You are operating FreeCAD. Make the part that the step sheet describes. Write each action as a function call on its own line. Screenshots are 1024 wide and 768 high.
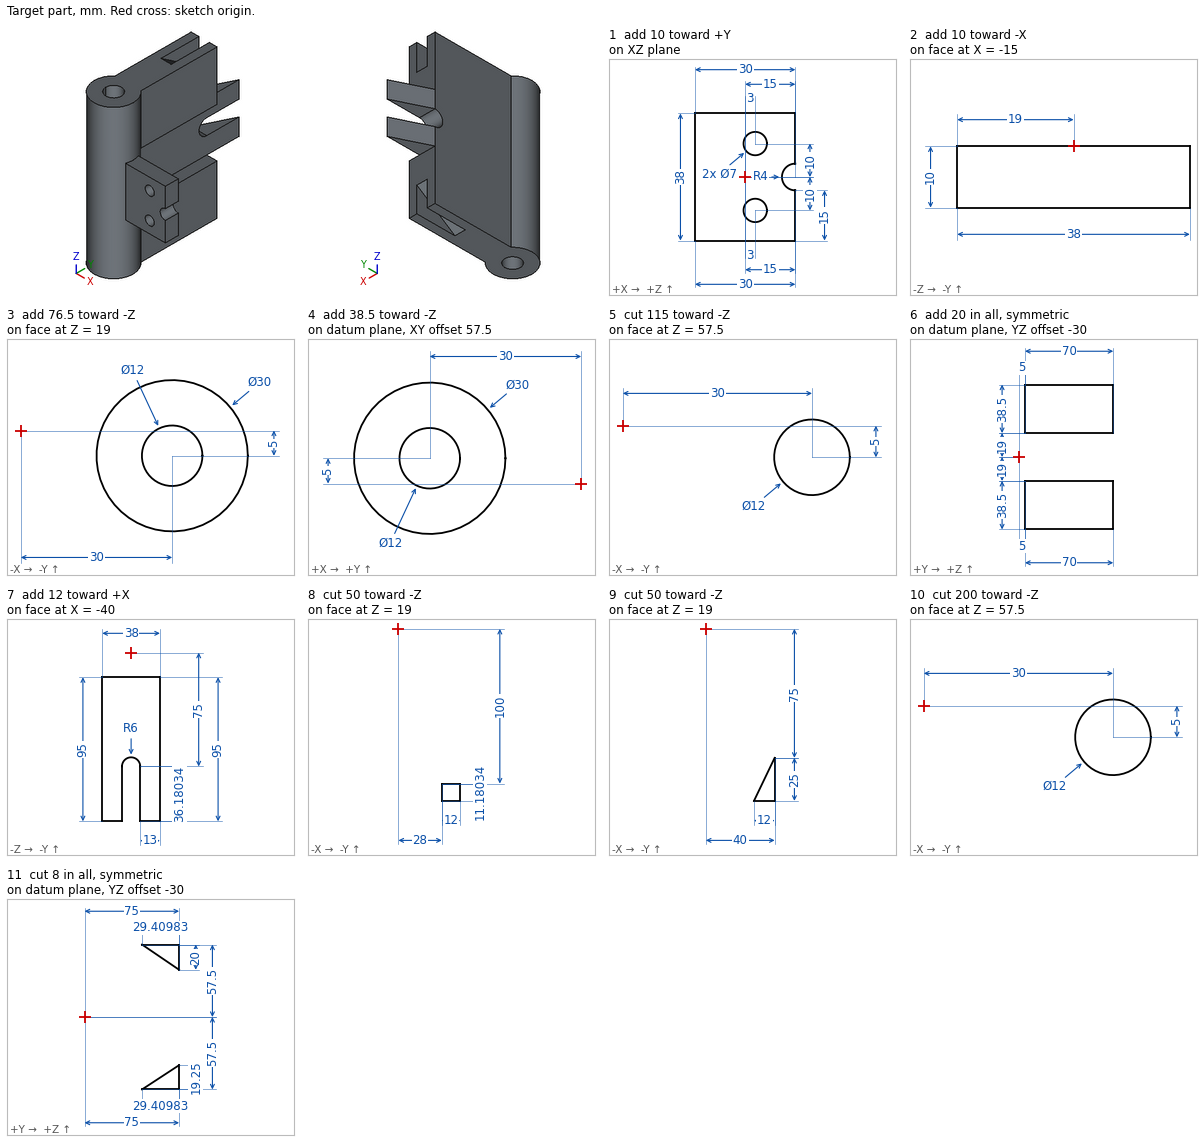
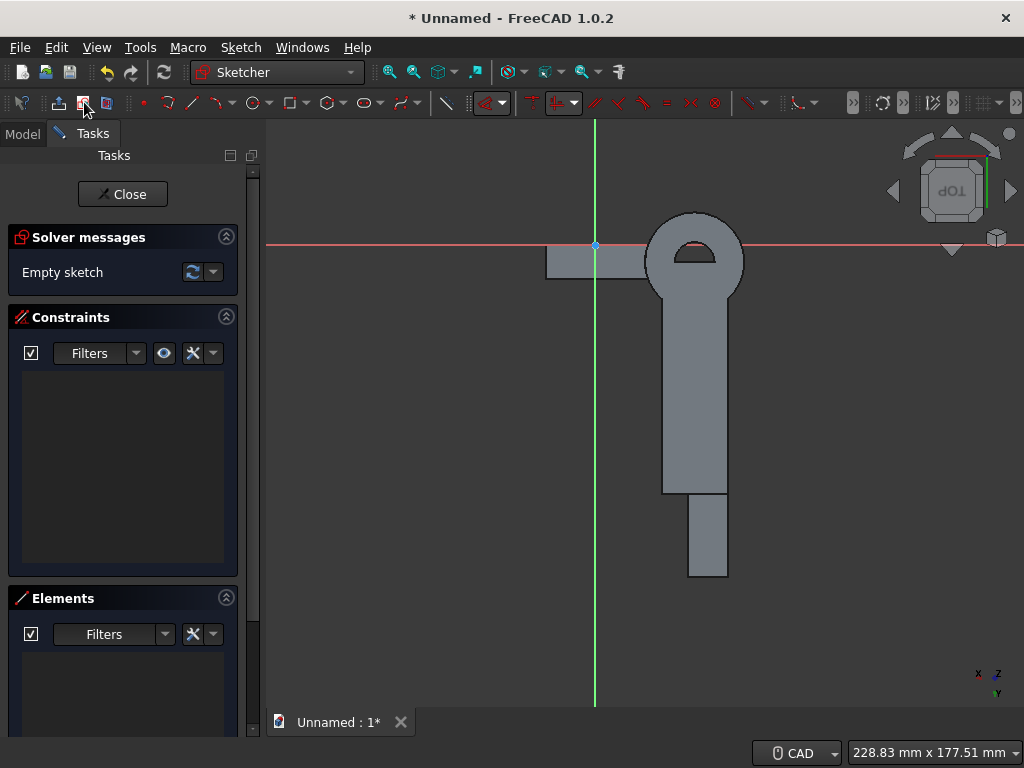
scroll(741, 566, up, 8)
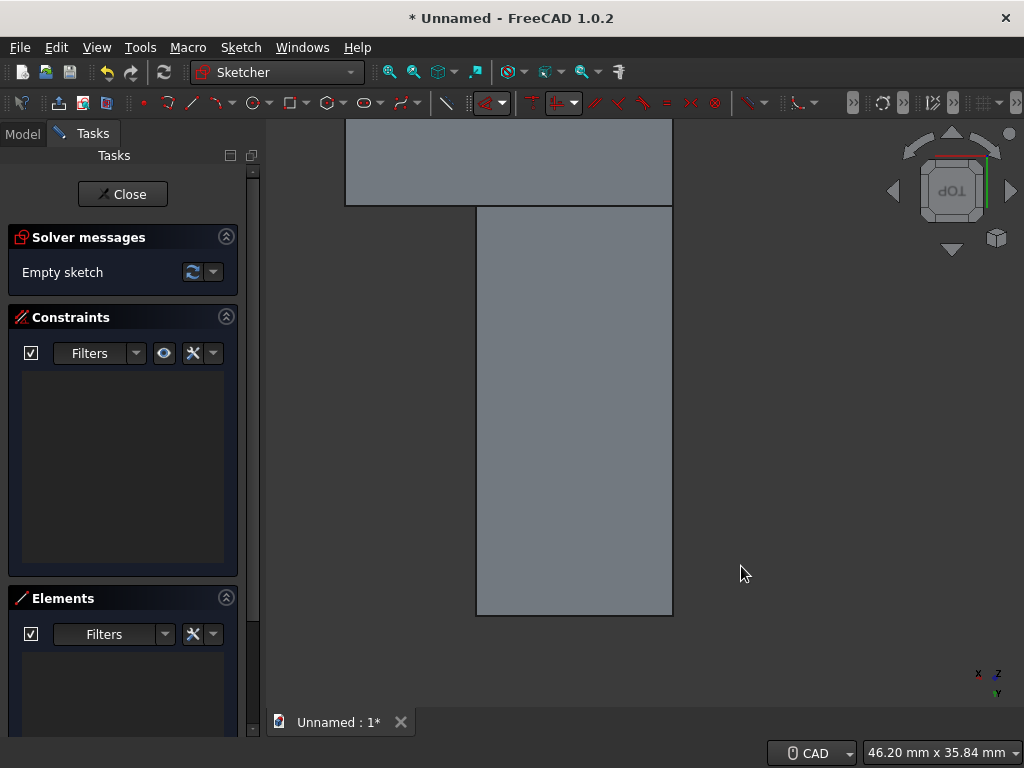
click(168, 104)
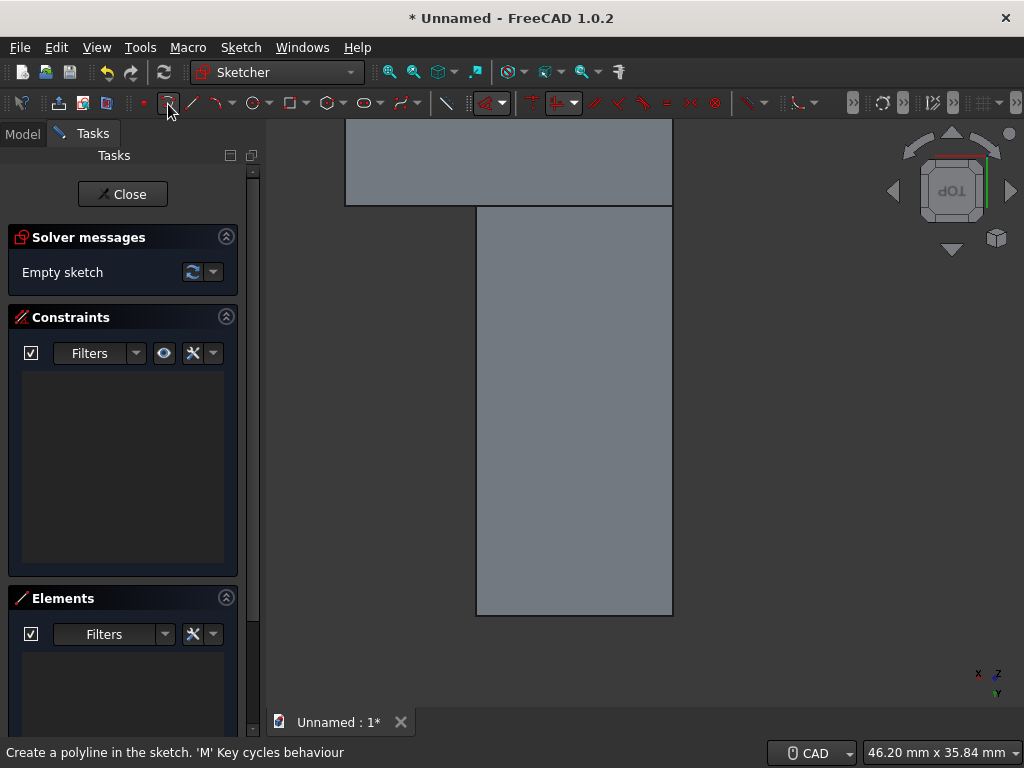
click(673, 206)
click(476, 616)
click(673, 616)
click(673, 207)
key(Escape)
key(Escape)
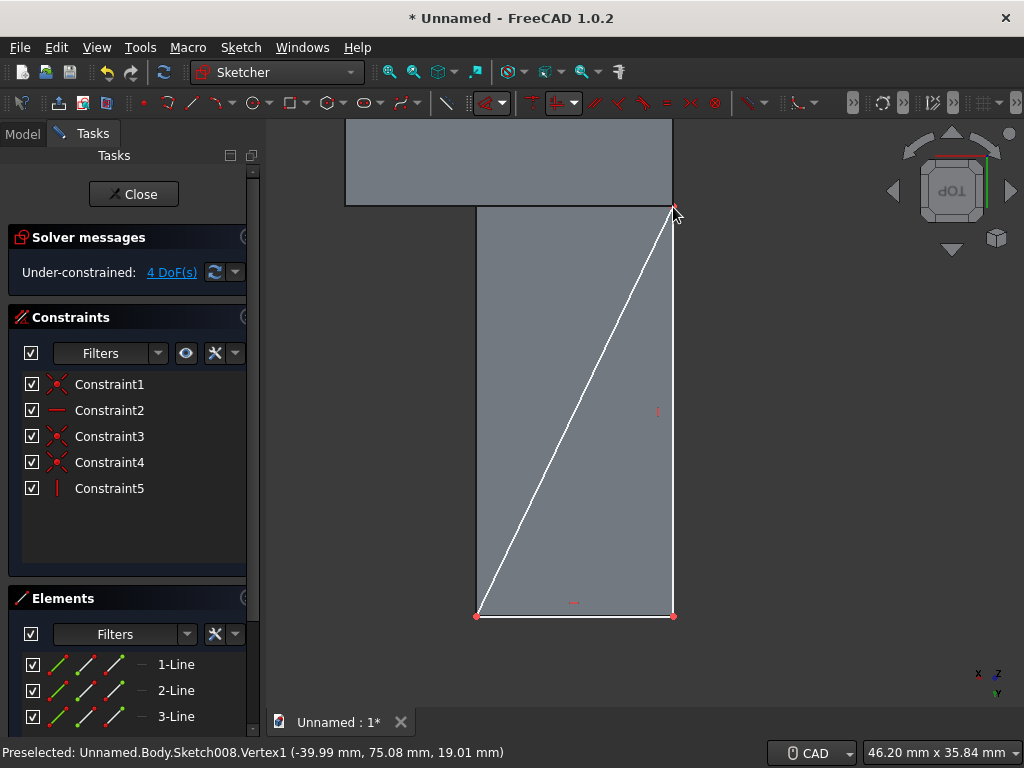
click(535, 617)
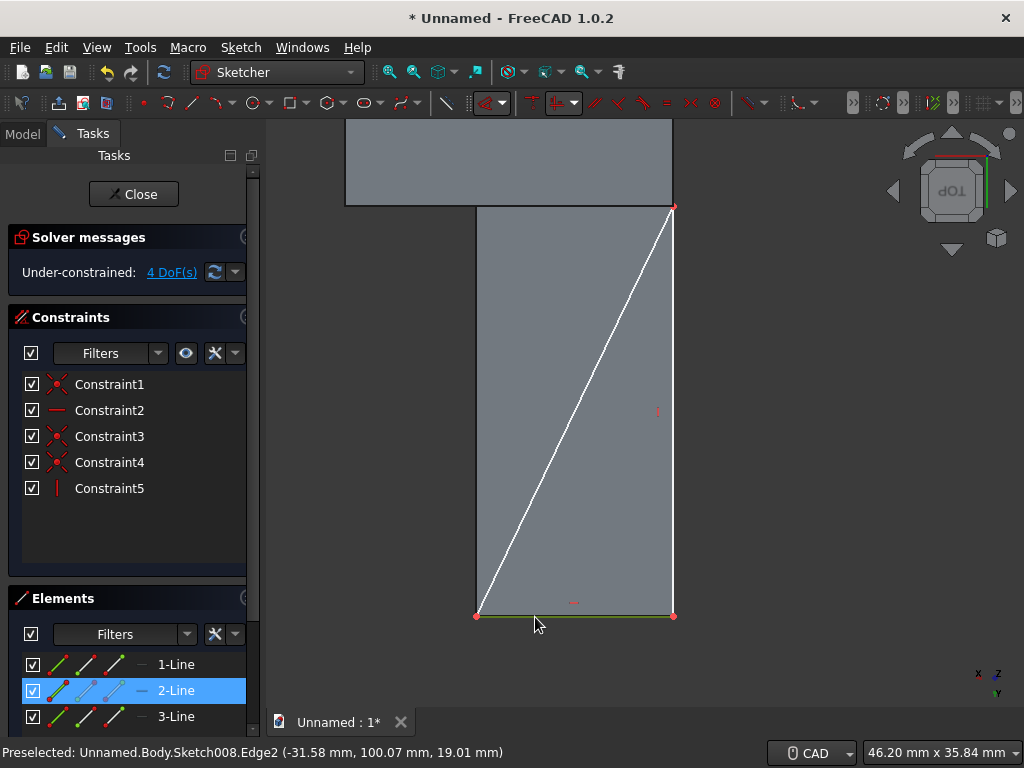
click(504, 104)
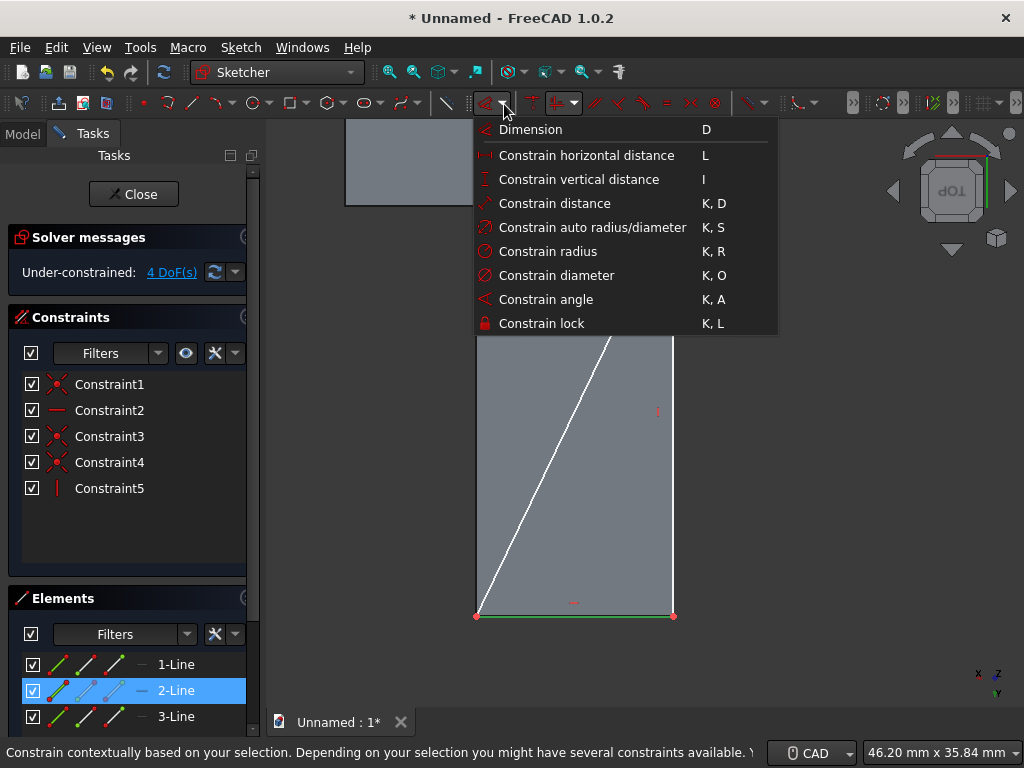
click(626, 155)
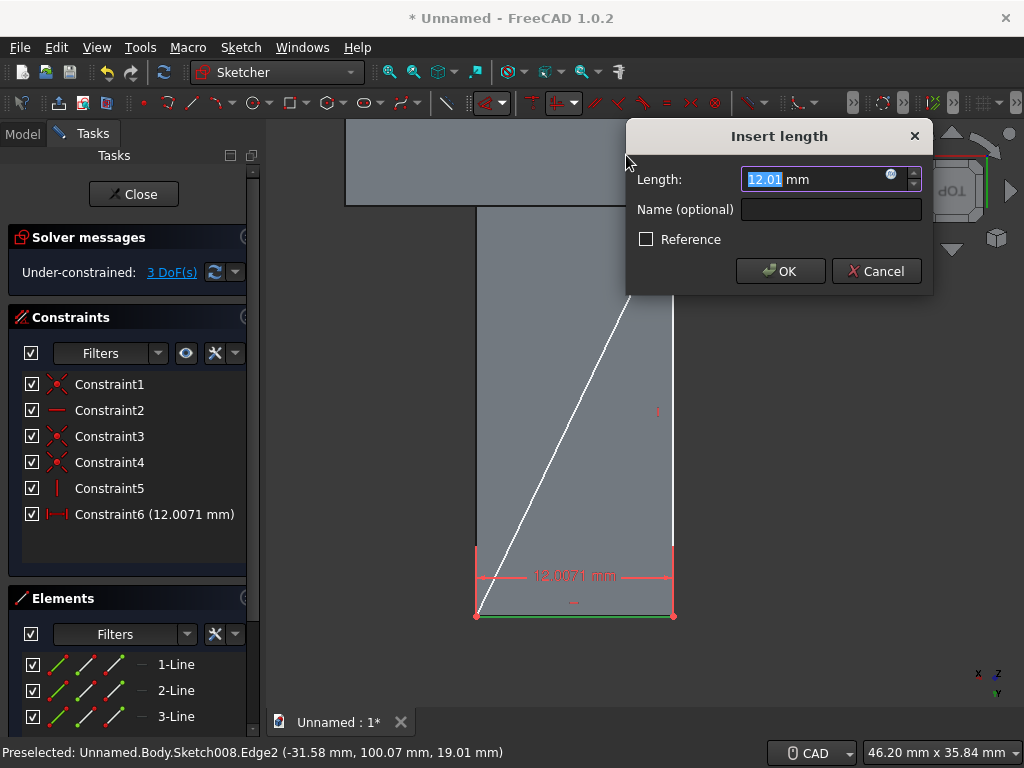
text(12)
key(Return)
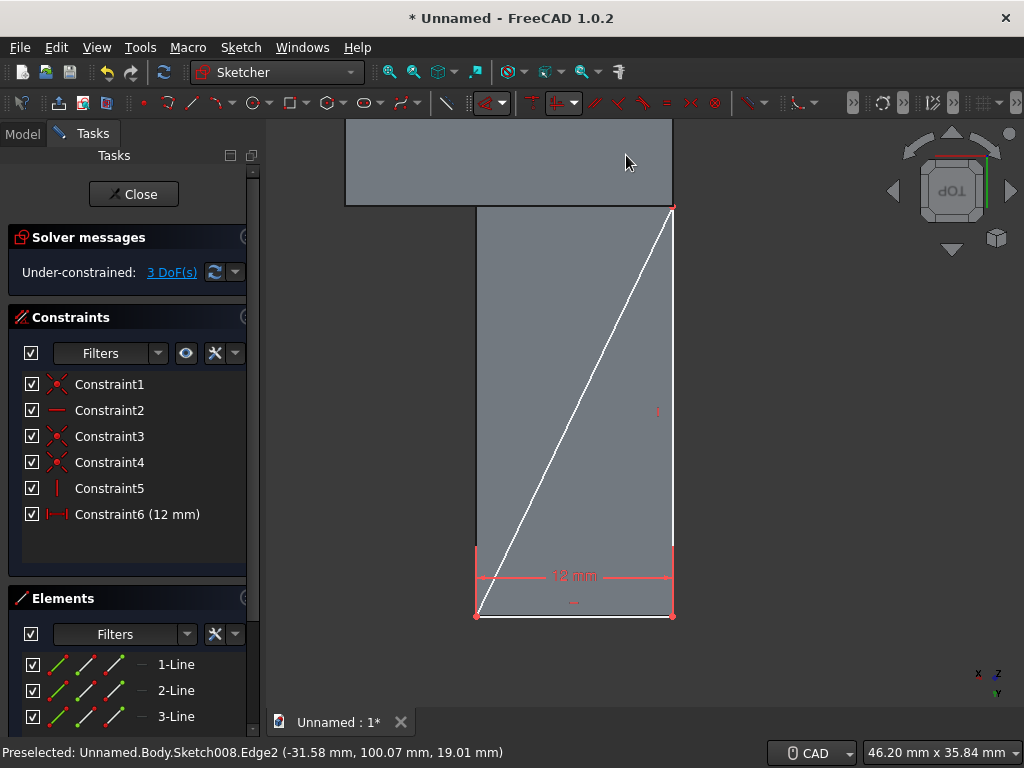
click(673, 494)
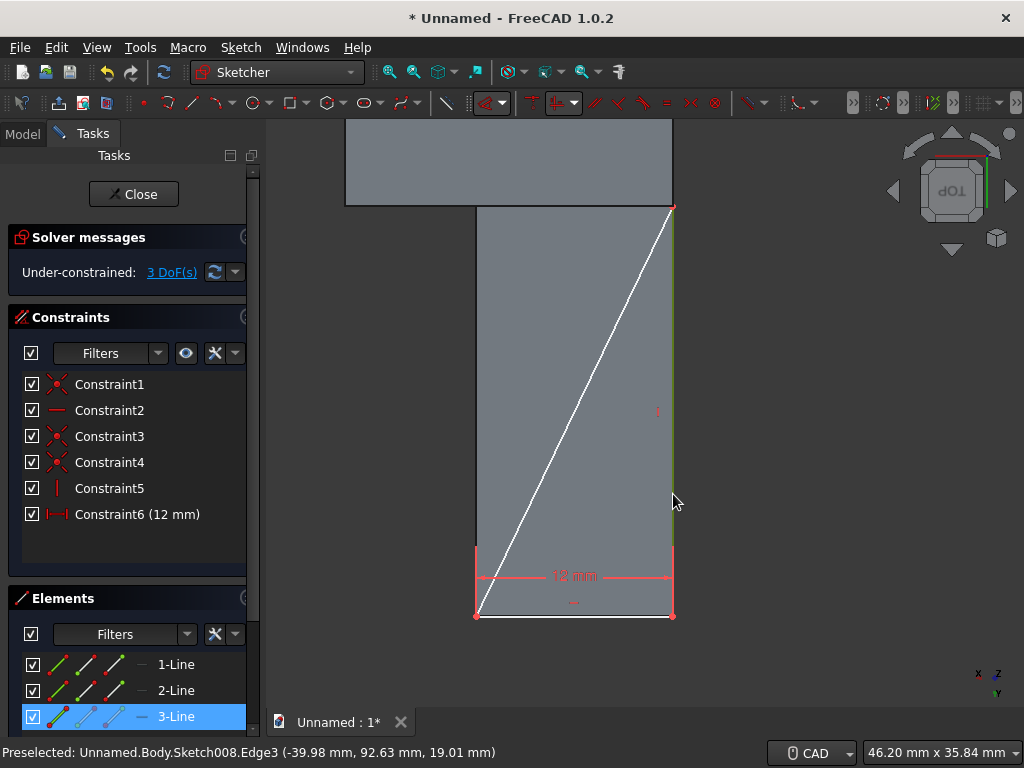
click(504, 104)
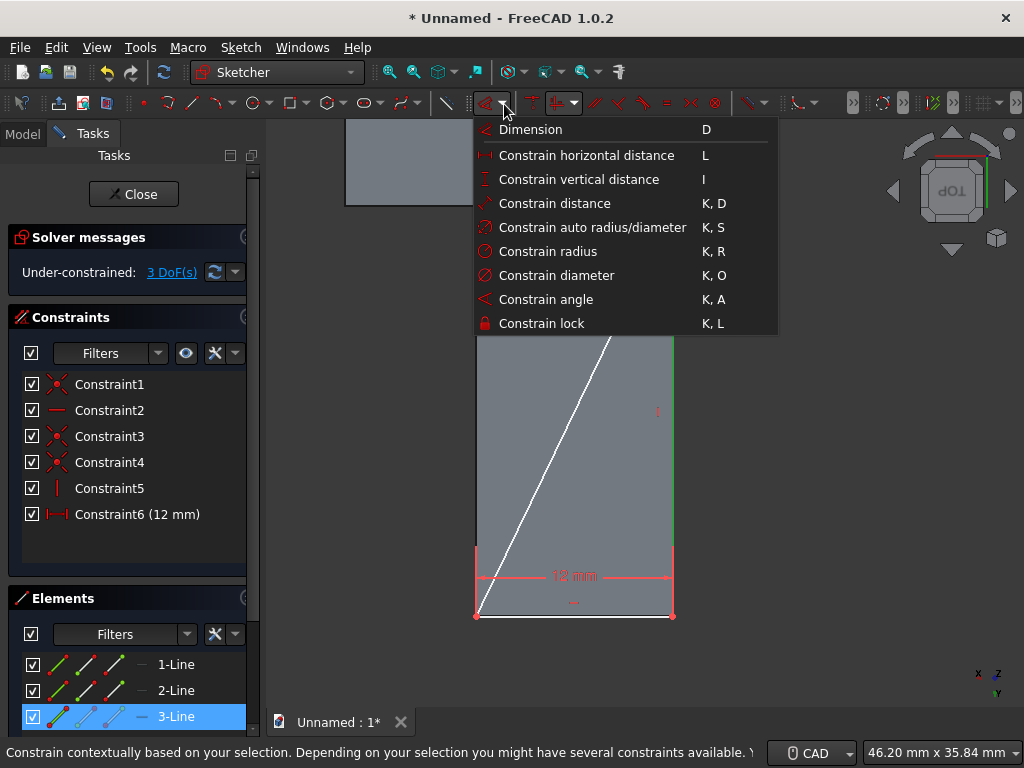
click(626, 179)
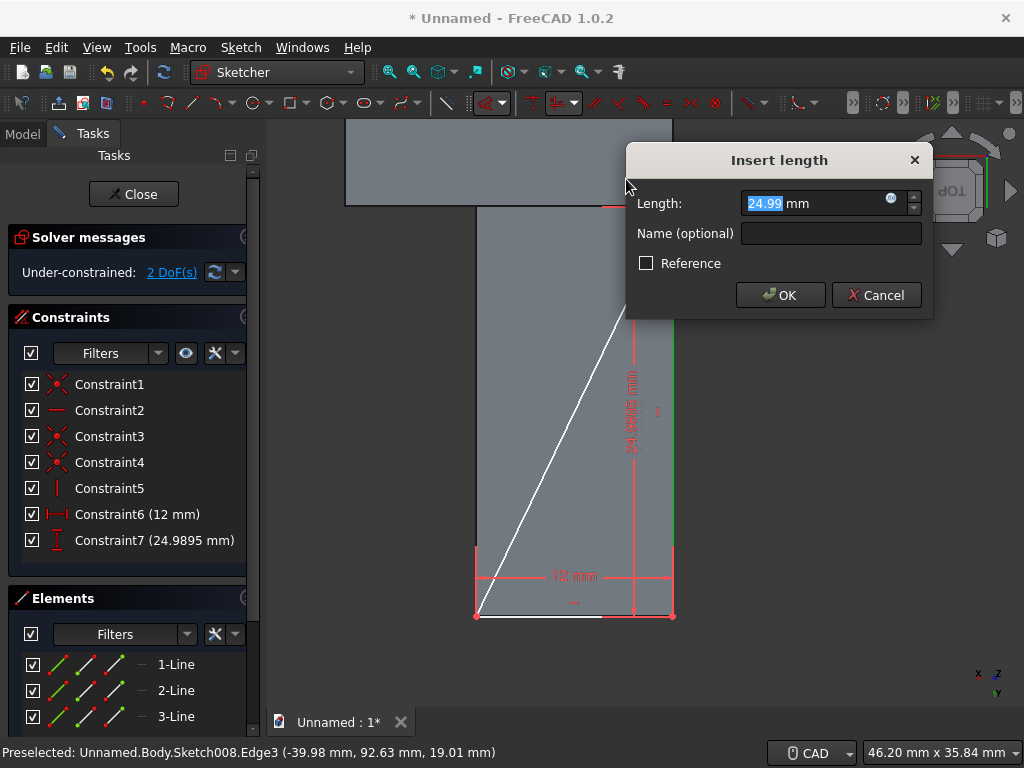
text(25)
key(Return)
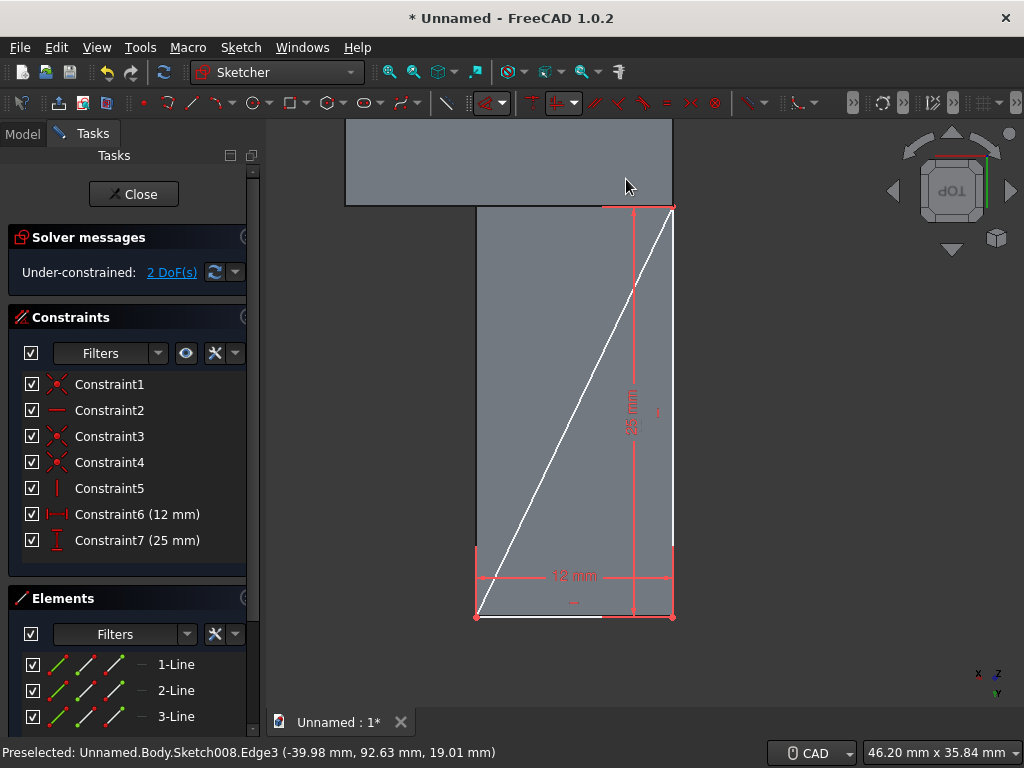
click(673, 207)